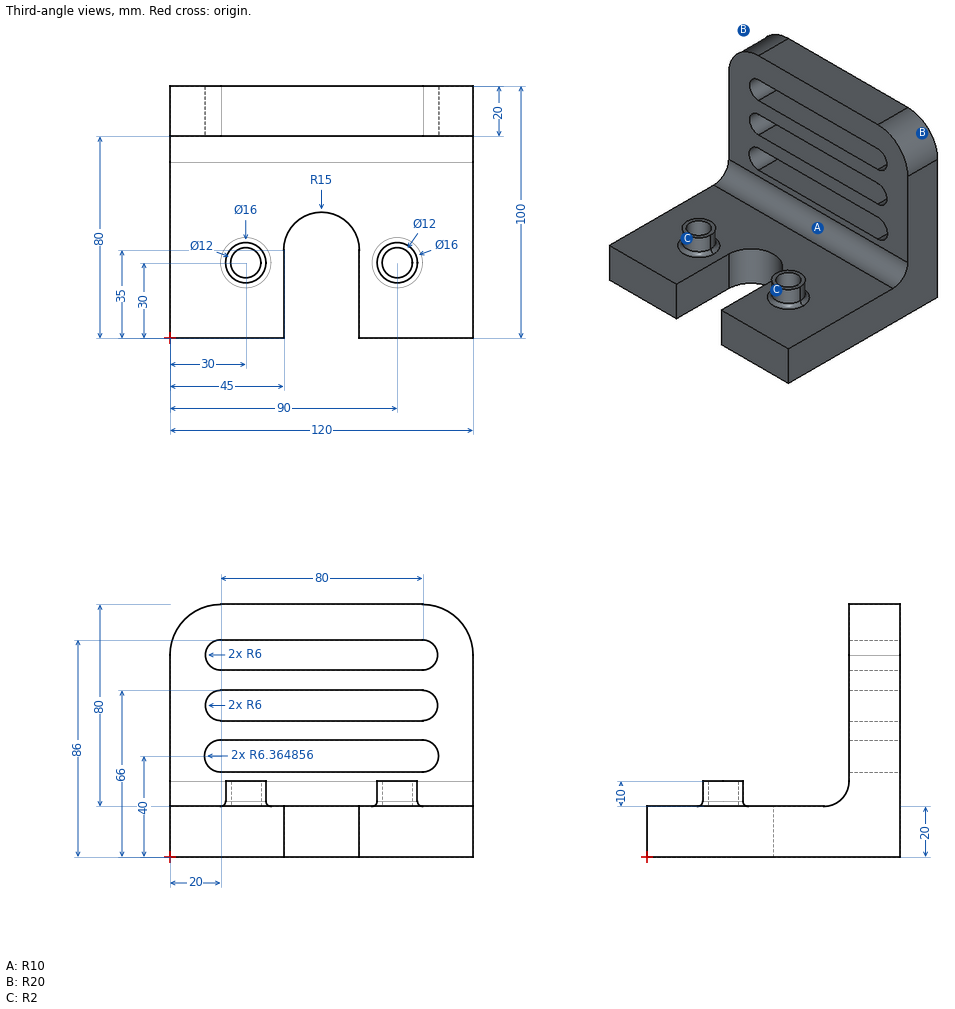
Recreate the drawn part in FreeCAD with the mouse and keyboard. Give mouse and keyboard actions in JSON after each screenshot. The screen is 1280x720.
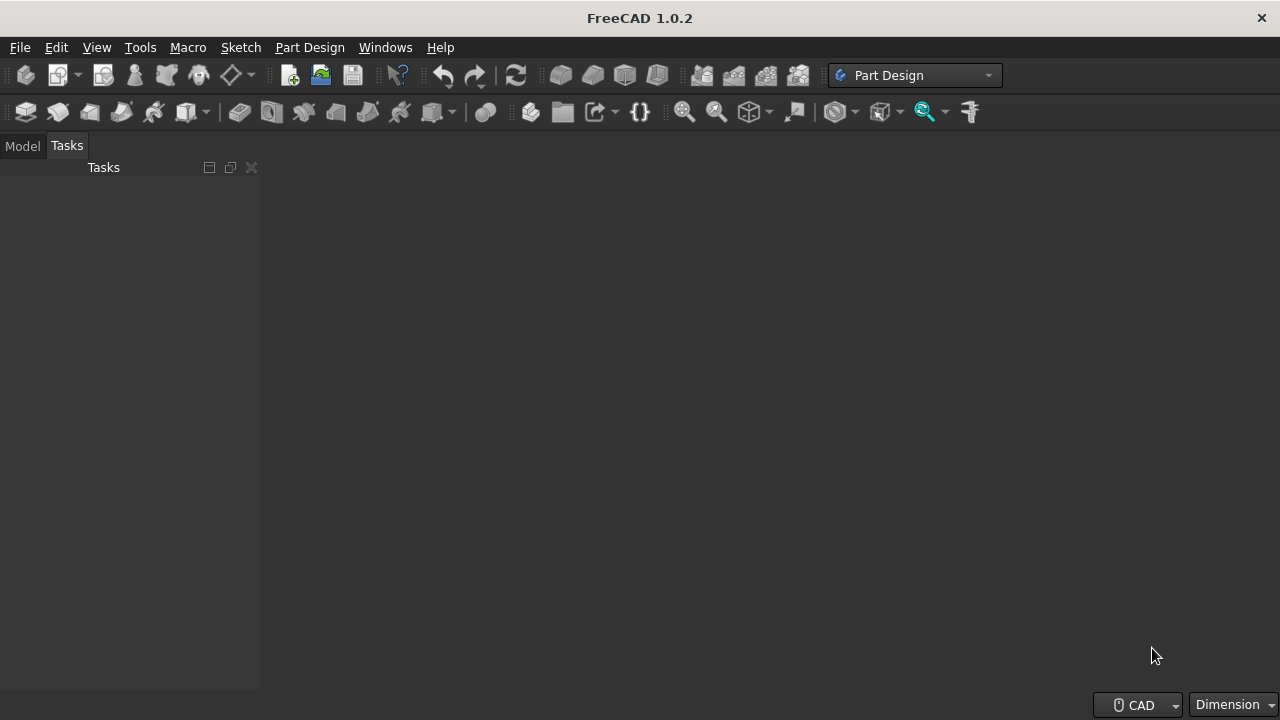
{"action": "left_click", "coordinate": [290, 76]}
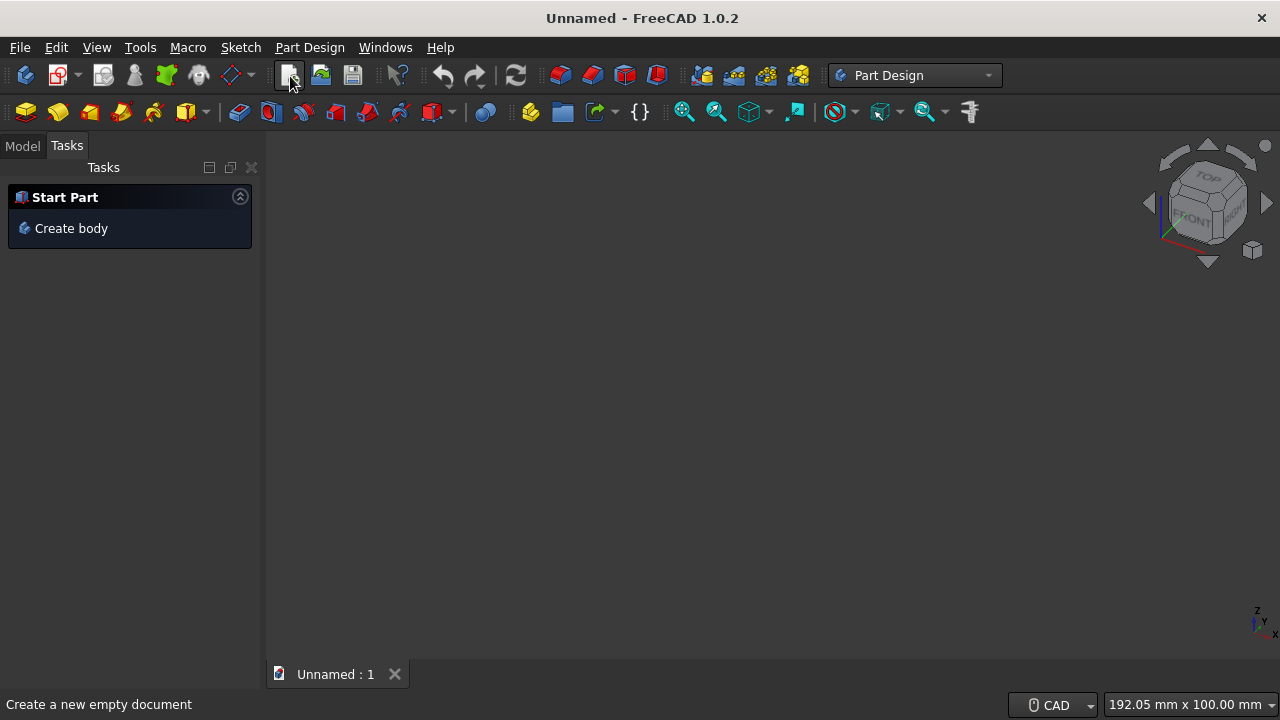
{"action": "left_click", "coordinate": [58, 76]}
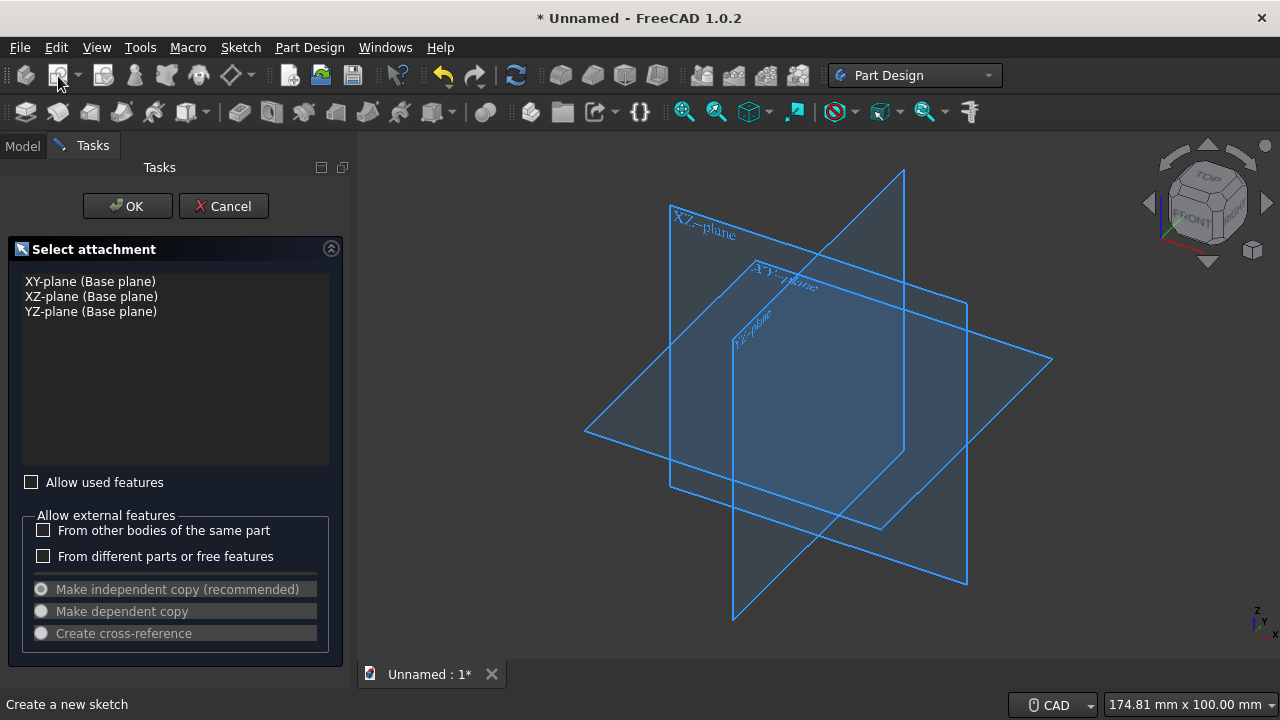
{"action": "left_click", "coordinate": [82, 282]}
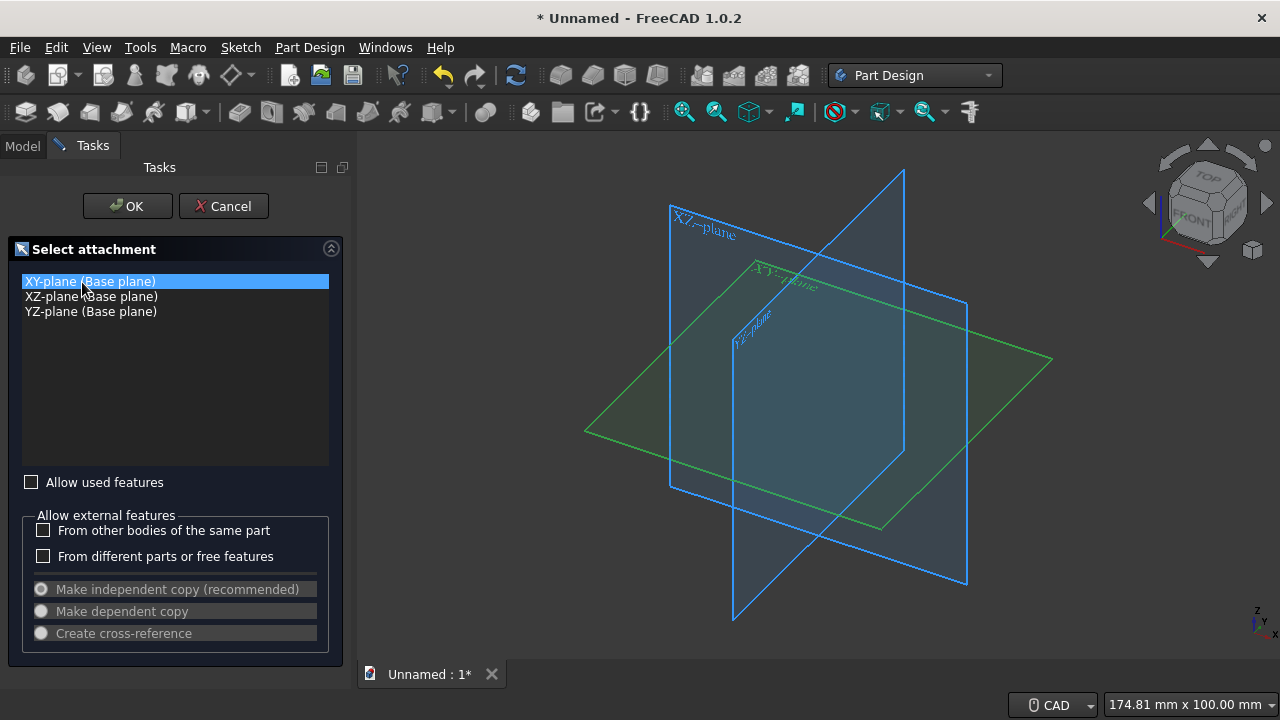
{"action": "left_click", "coordinate": [128, 206]}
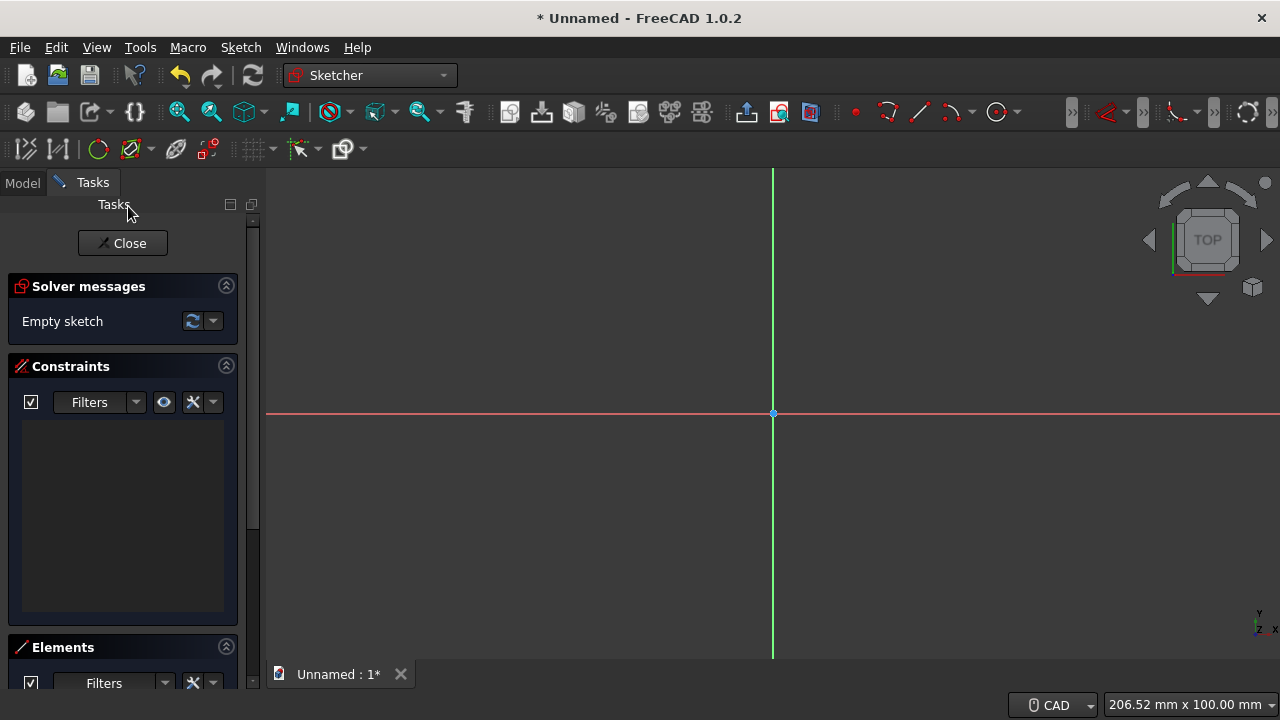
{"action": "scroll", "coordinate": [294, 631], "scroll_direction": "down", "scroll_amount": 3}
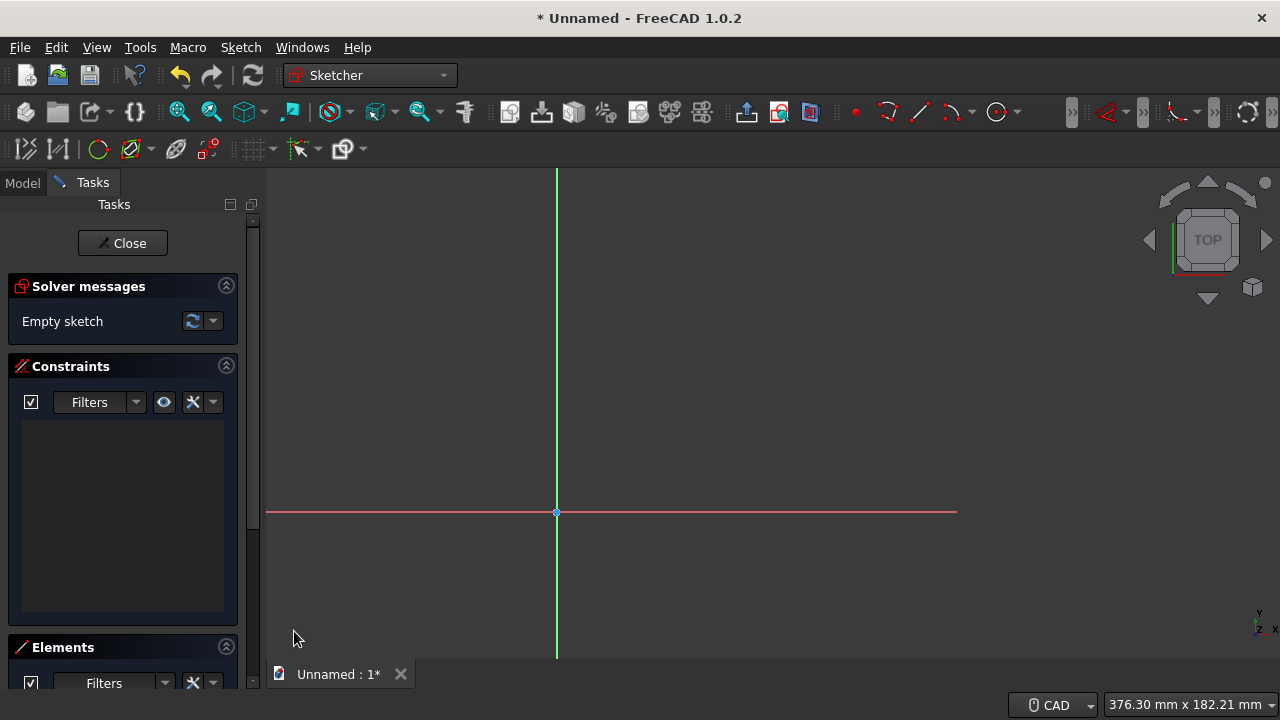
{"action": "key", "text": "g r"}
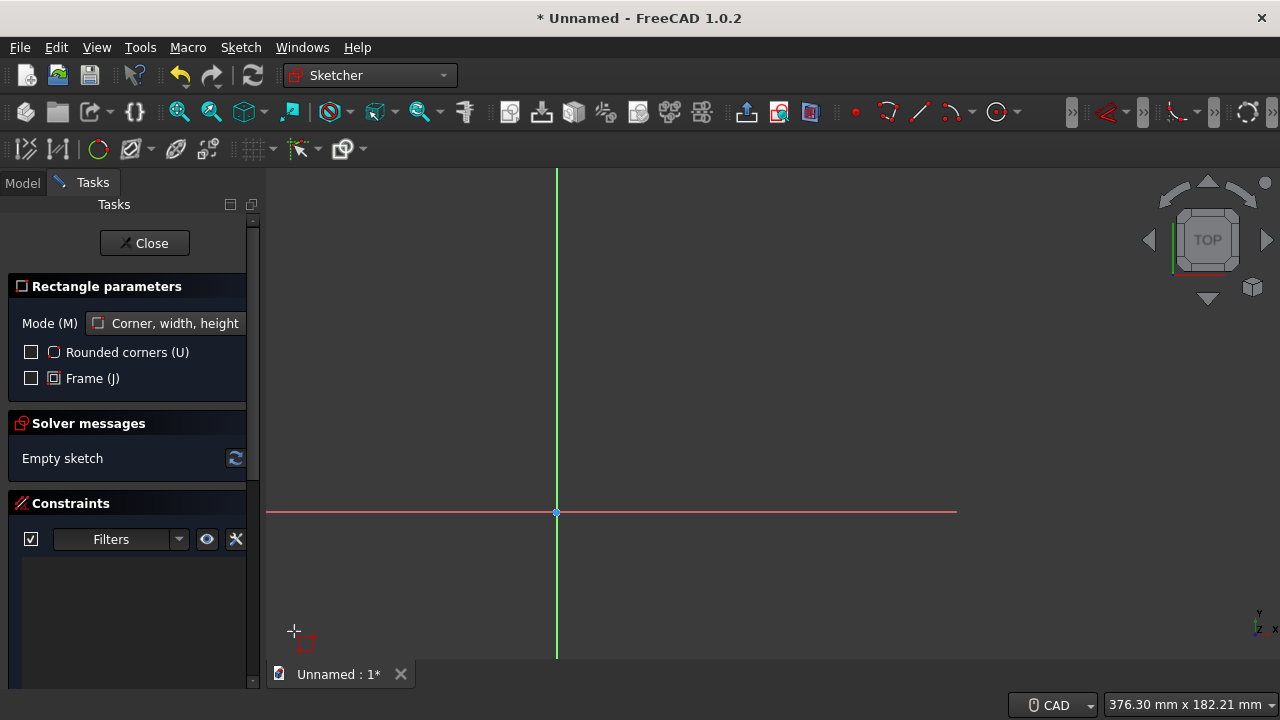
{"action": "left_click", "coordinate": [557, 512]}
{"action": "mouse_move", "coordinate": [880, 243]}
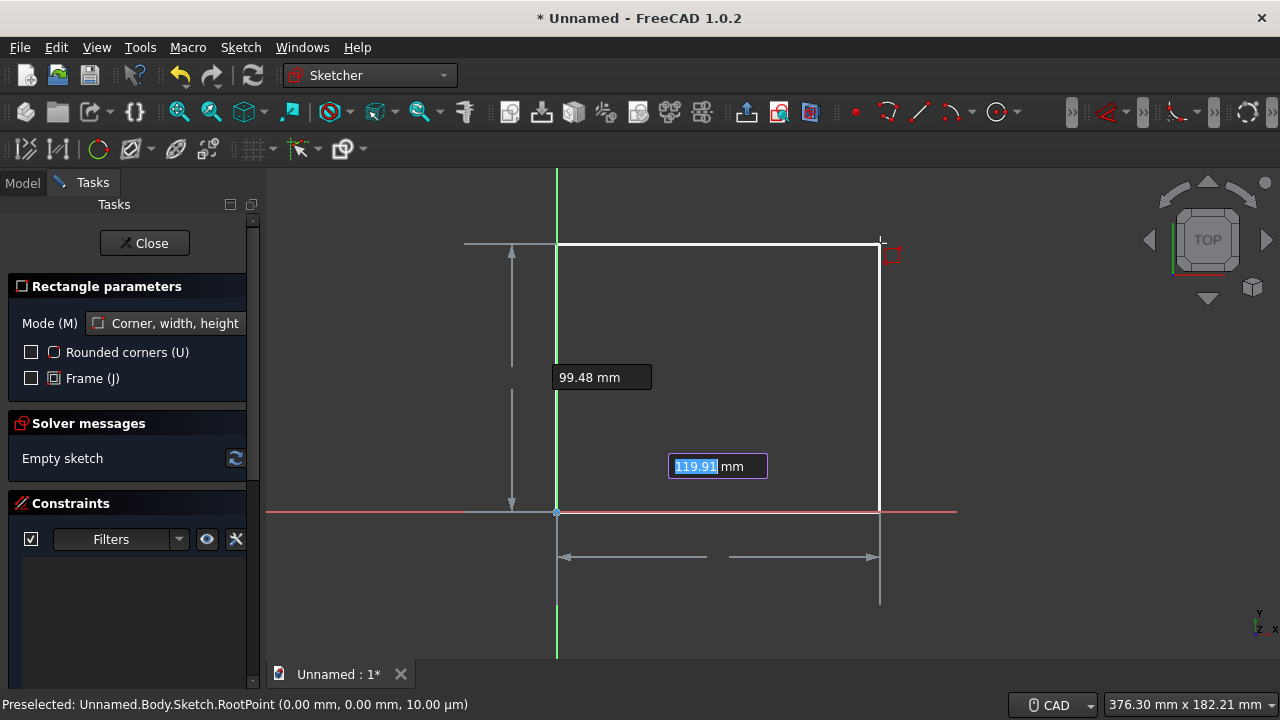
{"action": "type", "text": "120"}
{"action": "key", "text": "Tab"}
{"action": "type", "text": "100"}
{"action": "key", "text": "Return"}
{"action": "key", "text": "Escape"}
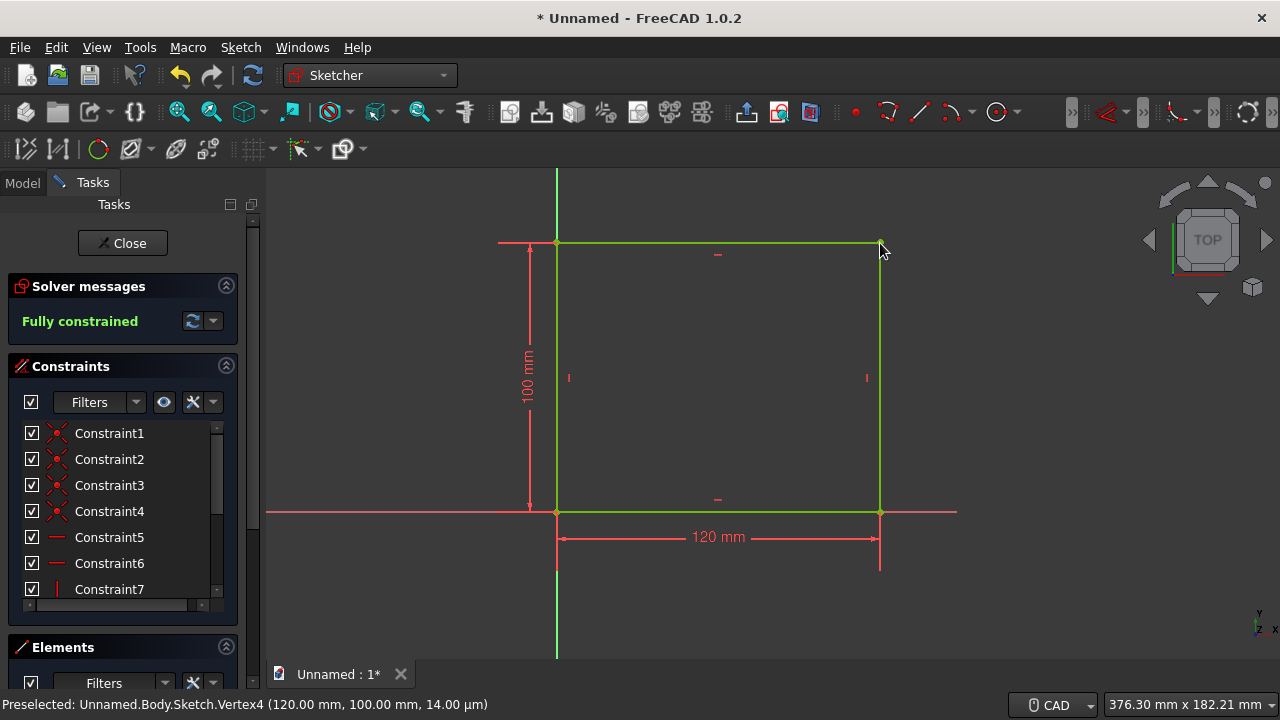
{"action": "left_click", "coordinate": [123, 243]}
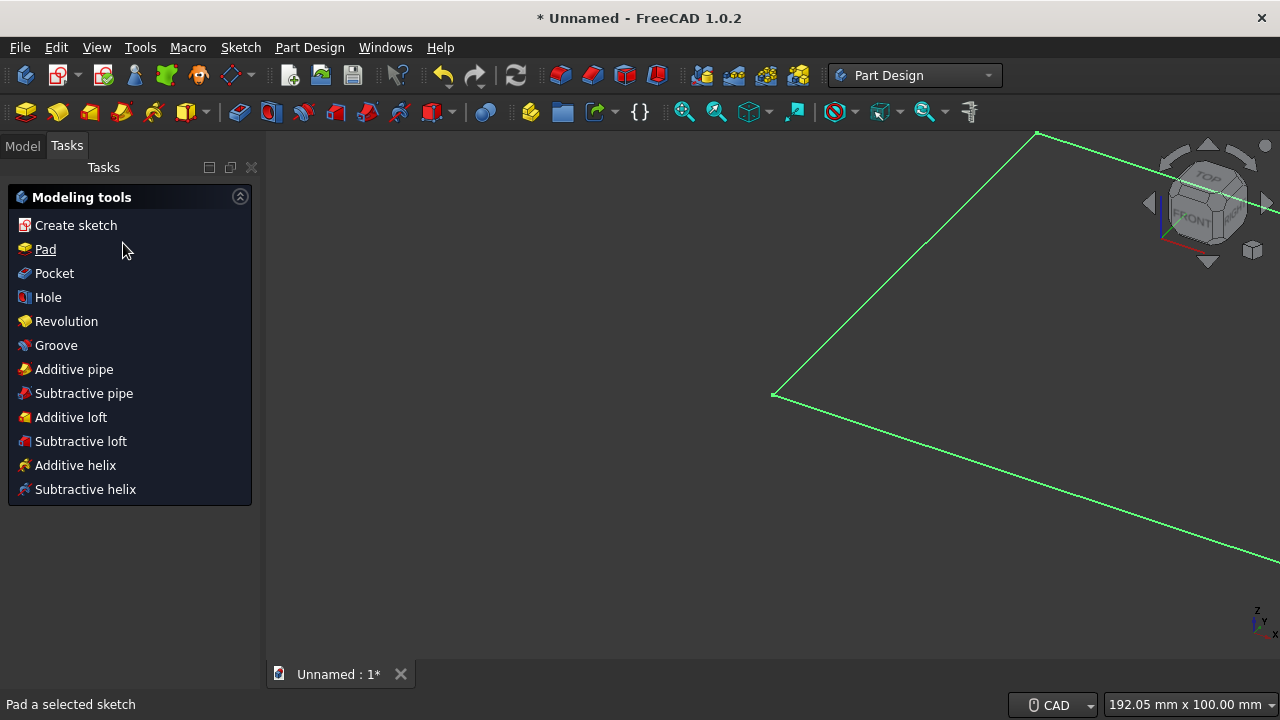
{"action": "left_click", "coordinate": [26, 112]}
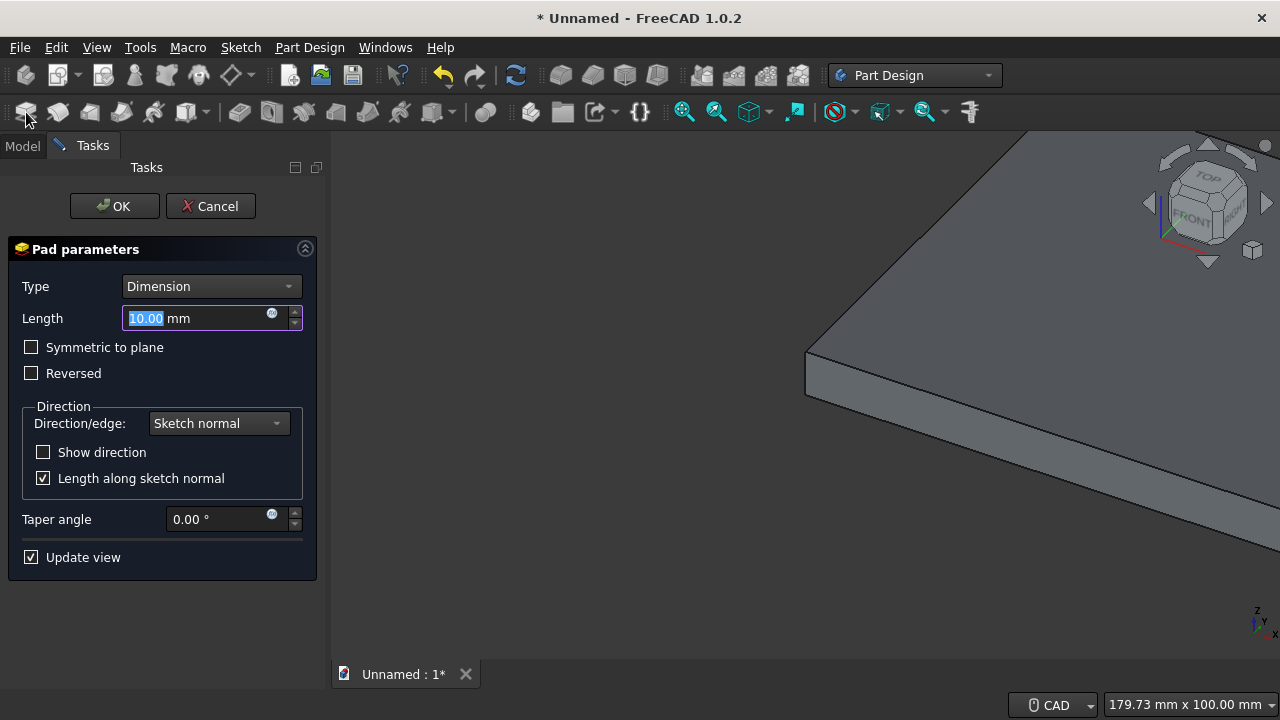
{"action": "type", "text": "20"}
{"action": "key", "text": "Tab"}